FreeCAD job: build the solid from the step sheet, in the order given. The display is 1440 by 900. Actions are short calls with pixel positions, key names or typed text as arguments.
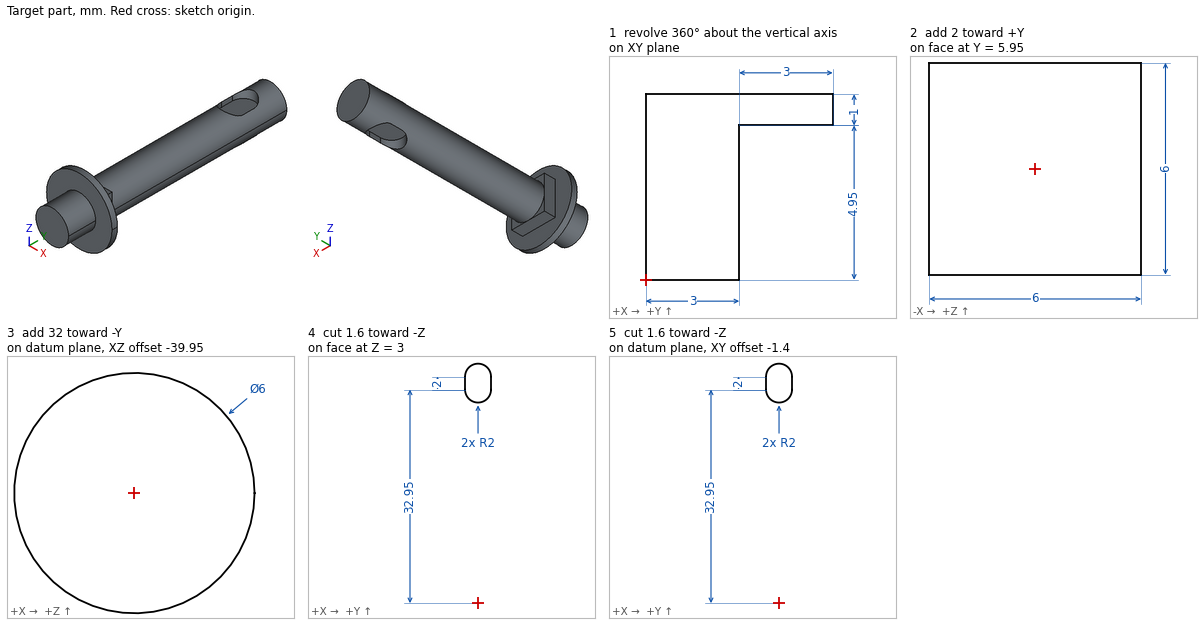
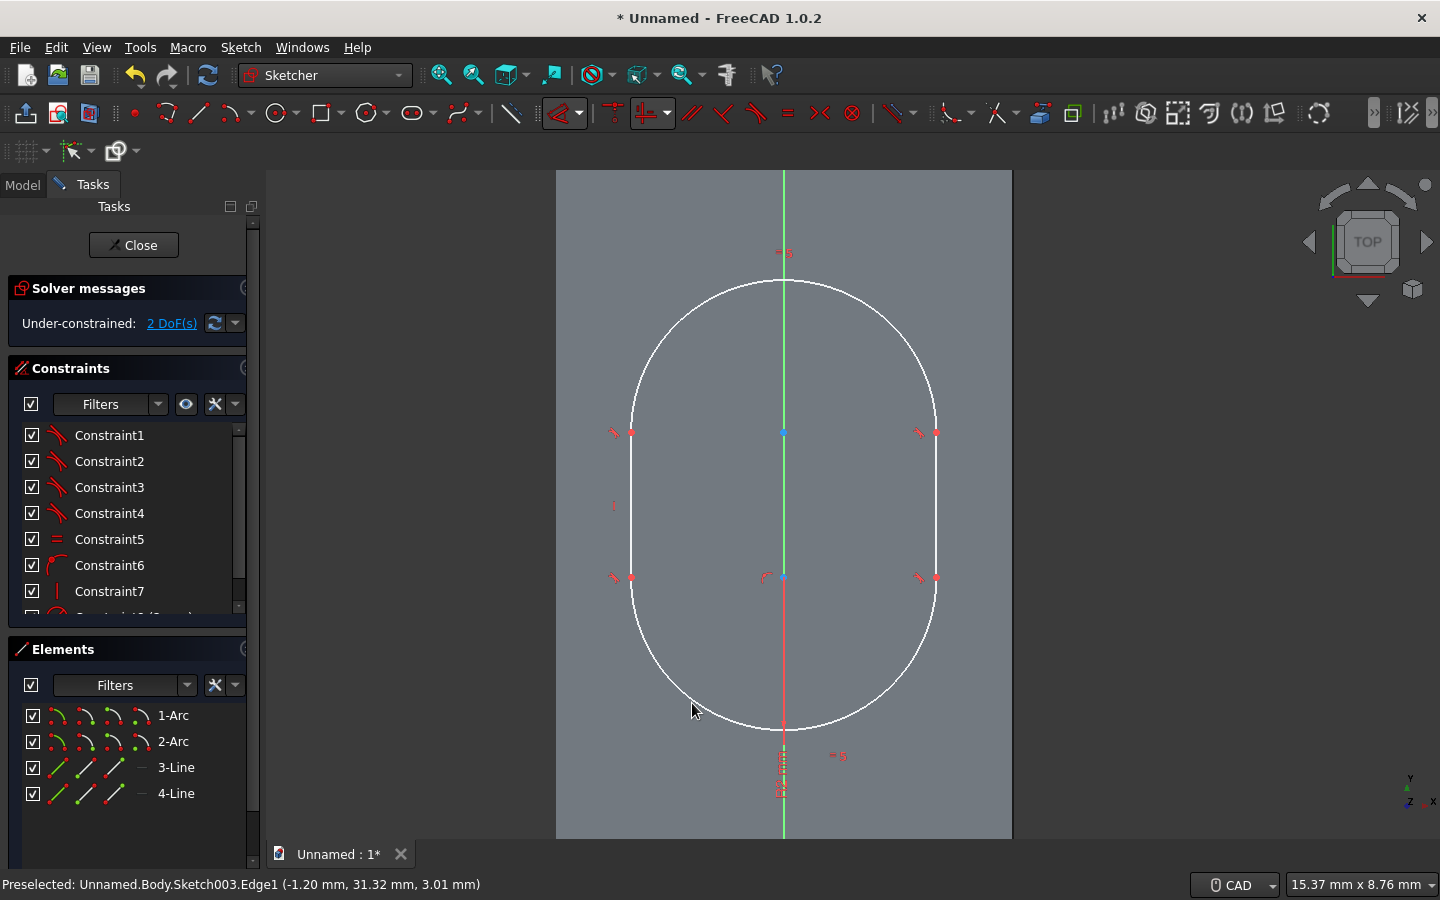
click(631, 534)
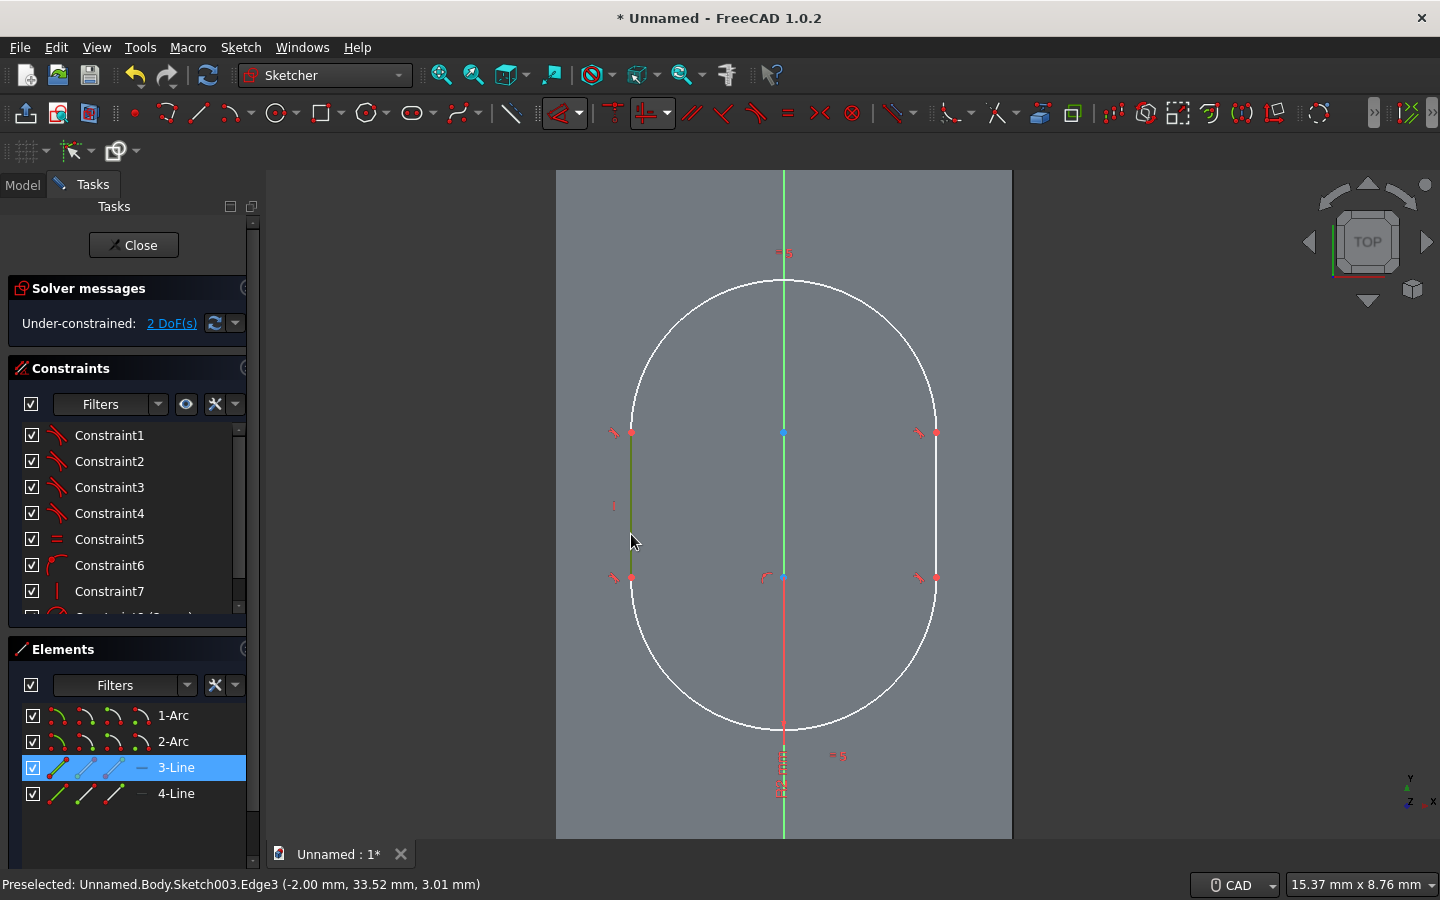
key(i)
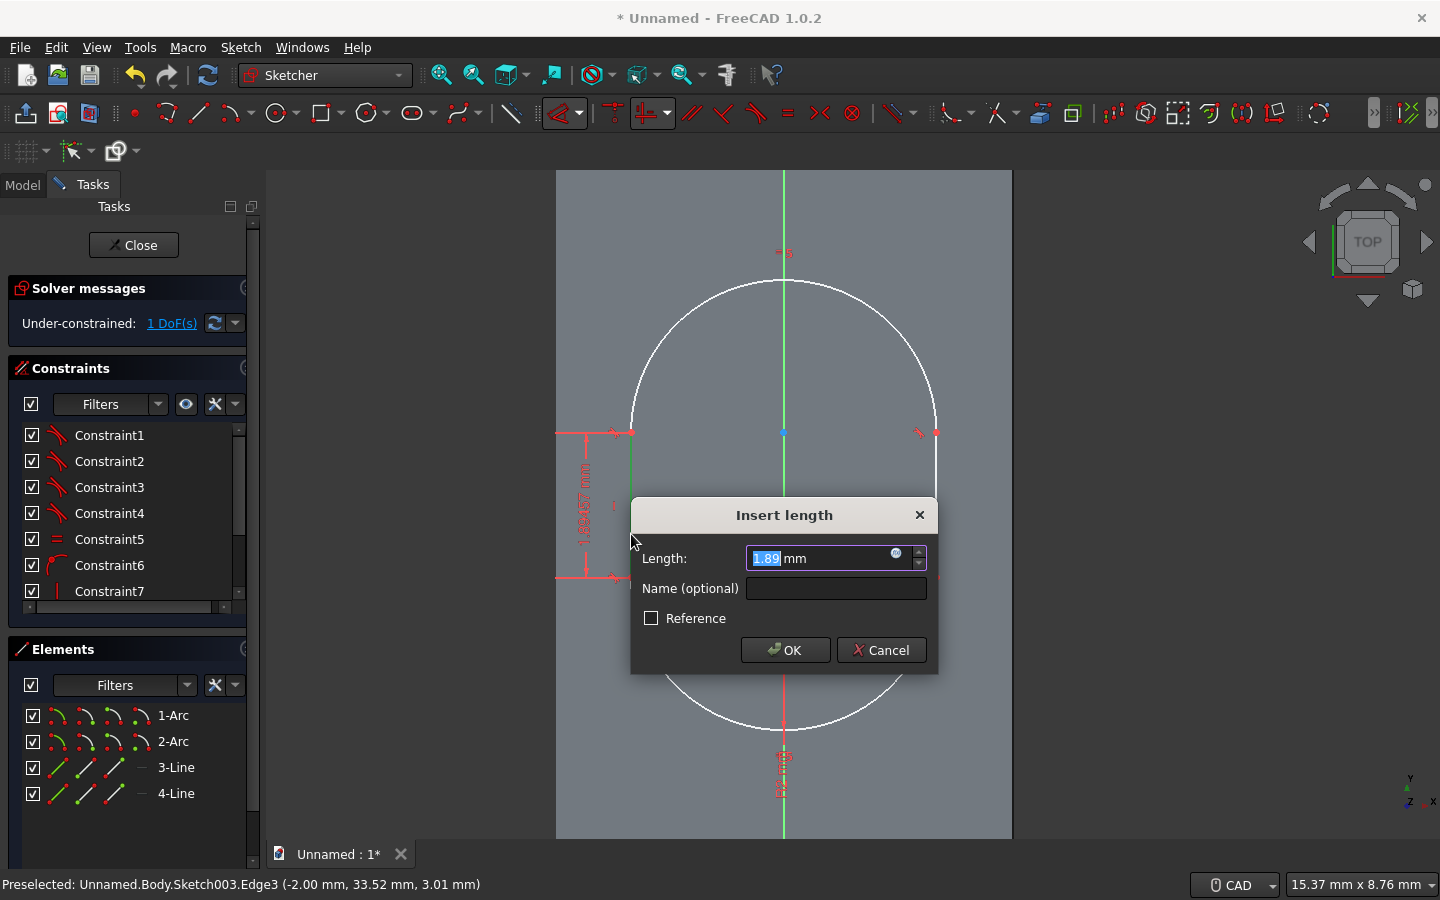
text(2)
key(Return)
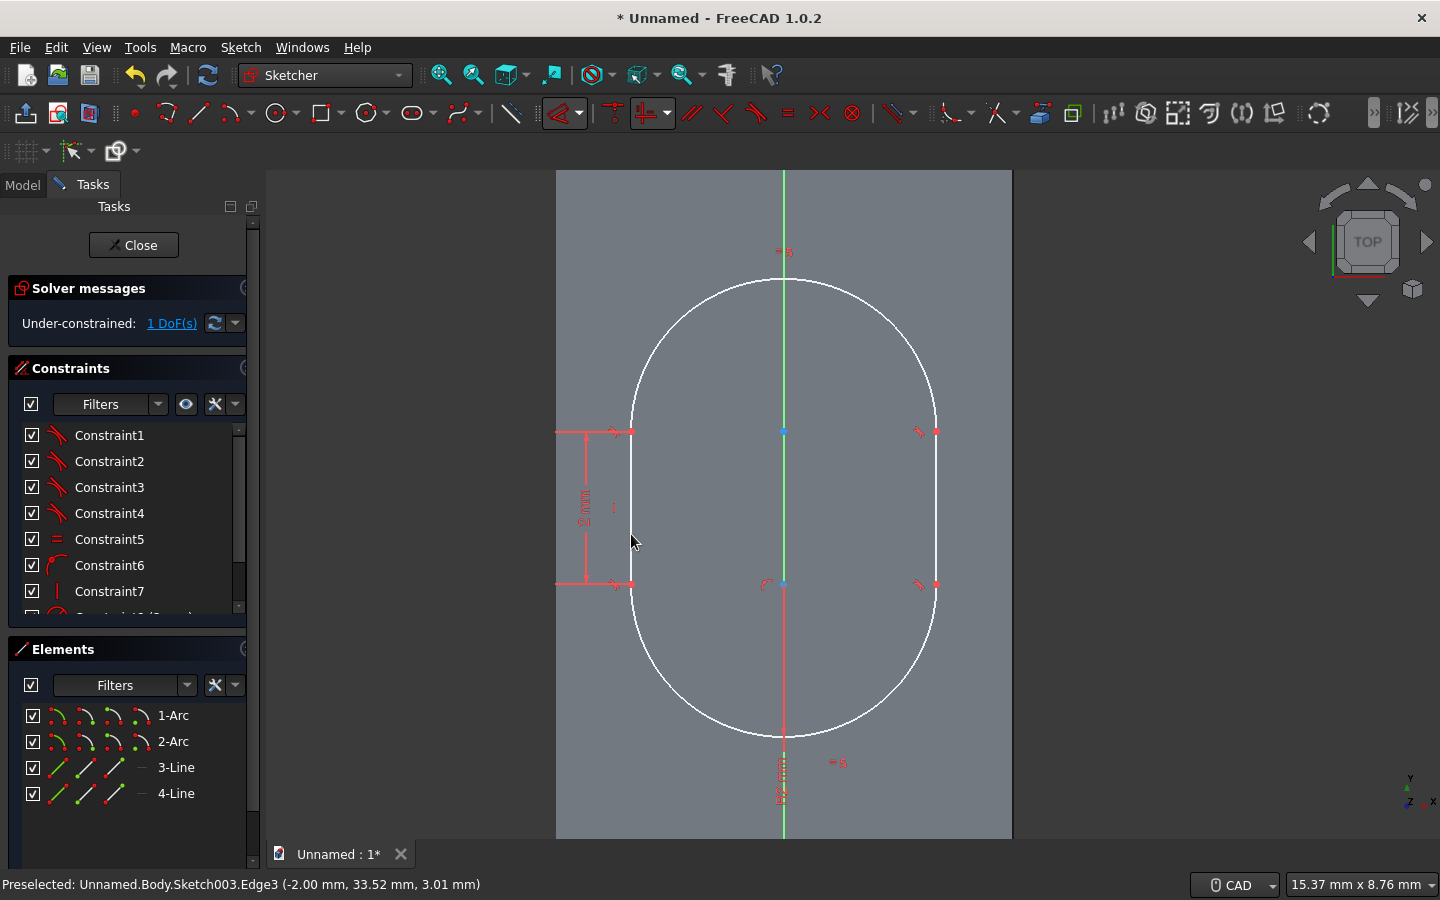
click(631, 584)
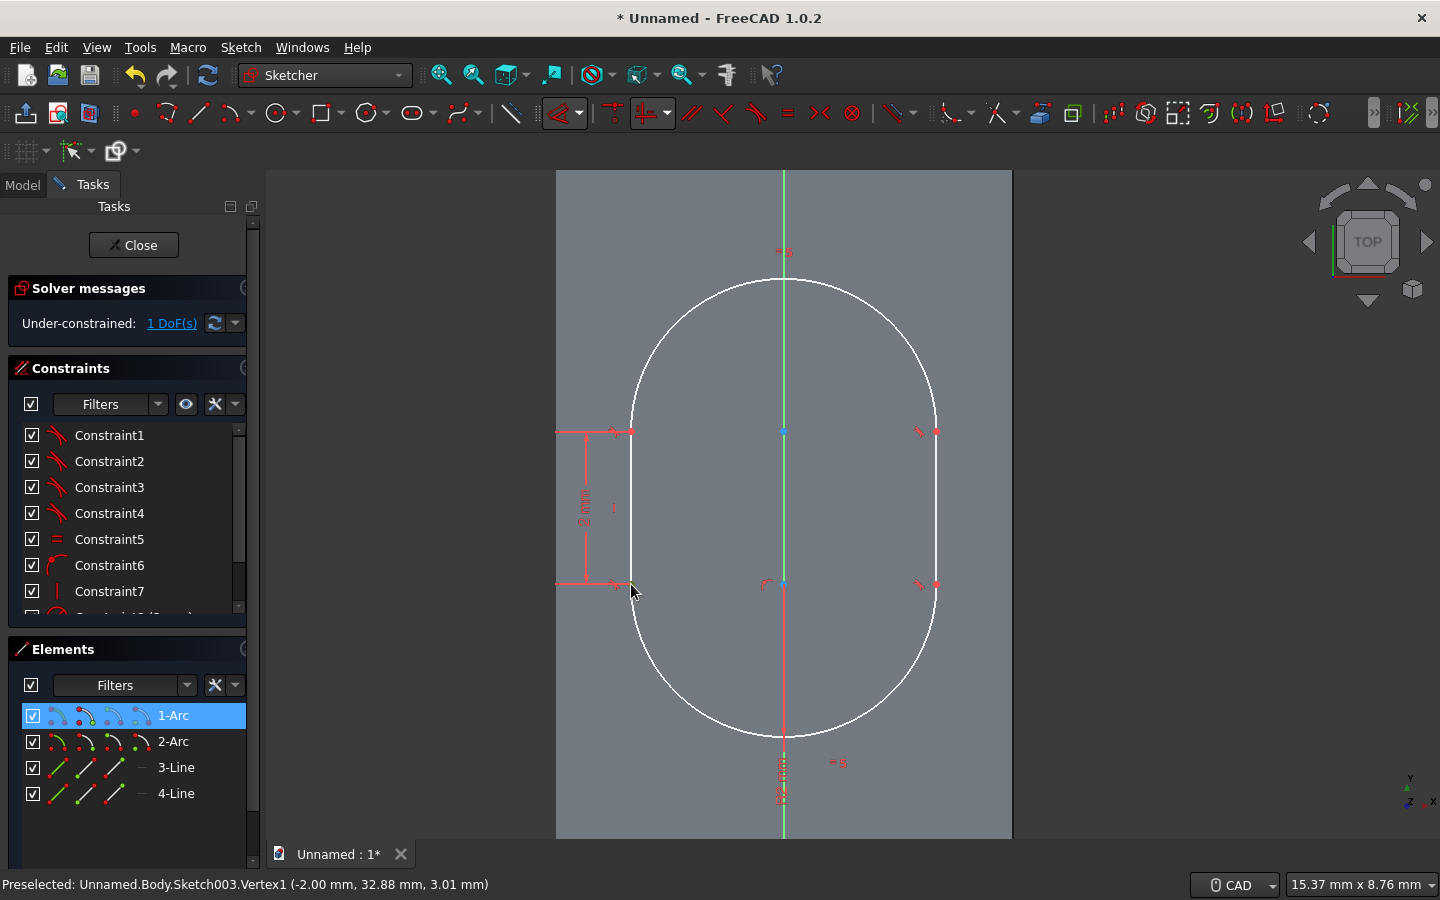
click(582, 114)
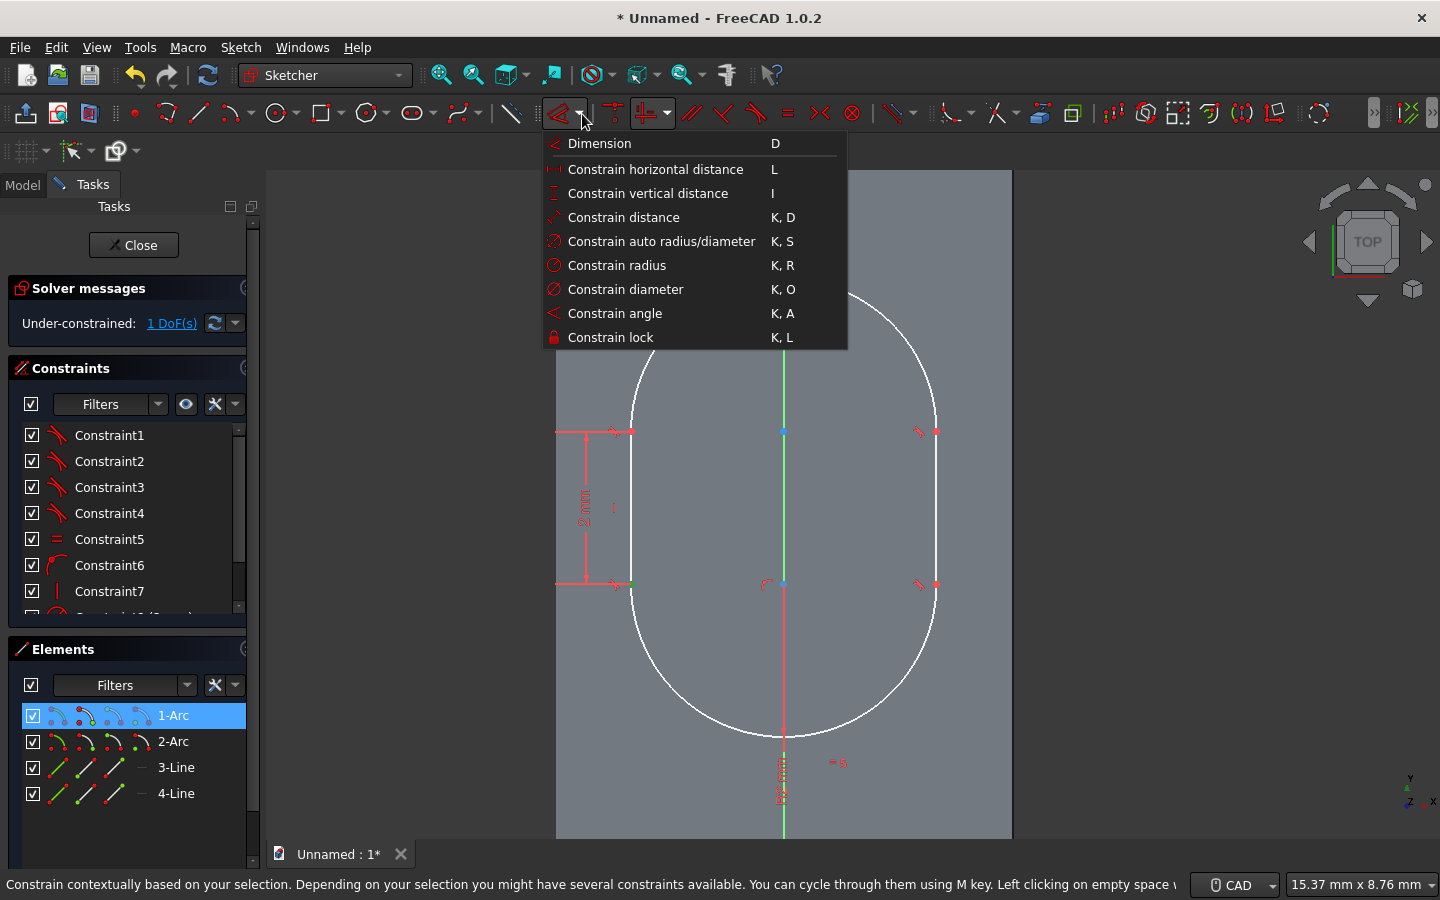
click(695, 193)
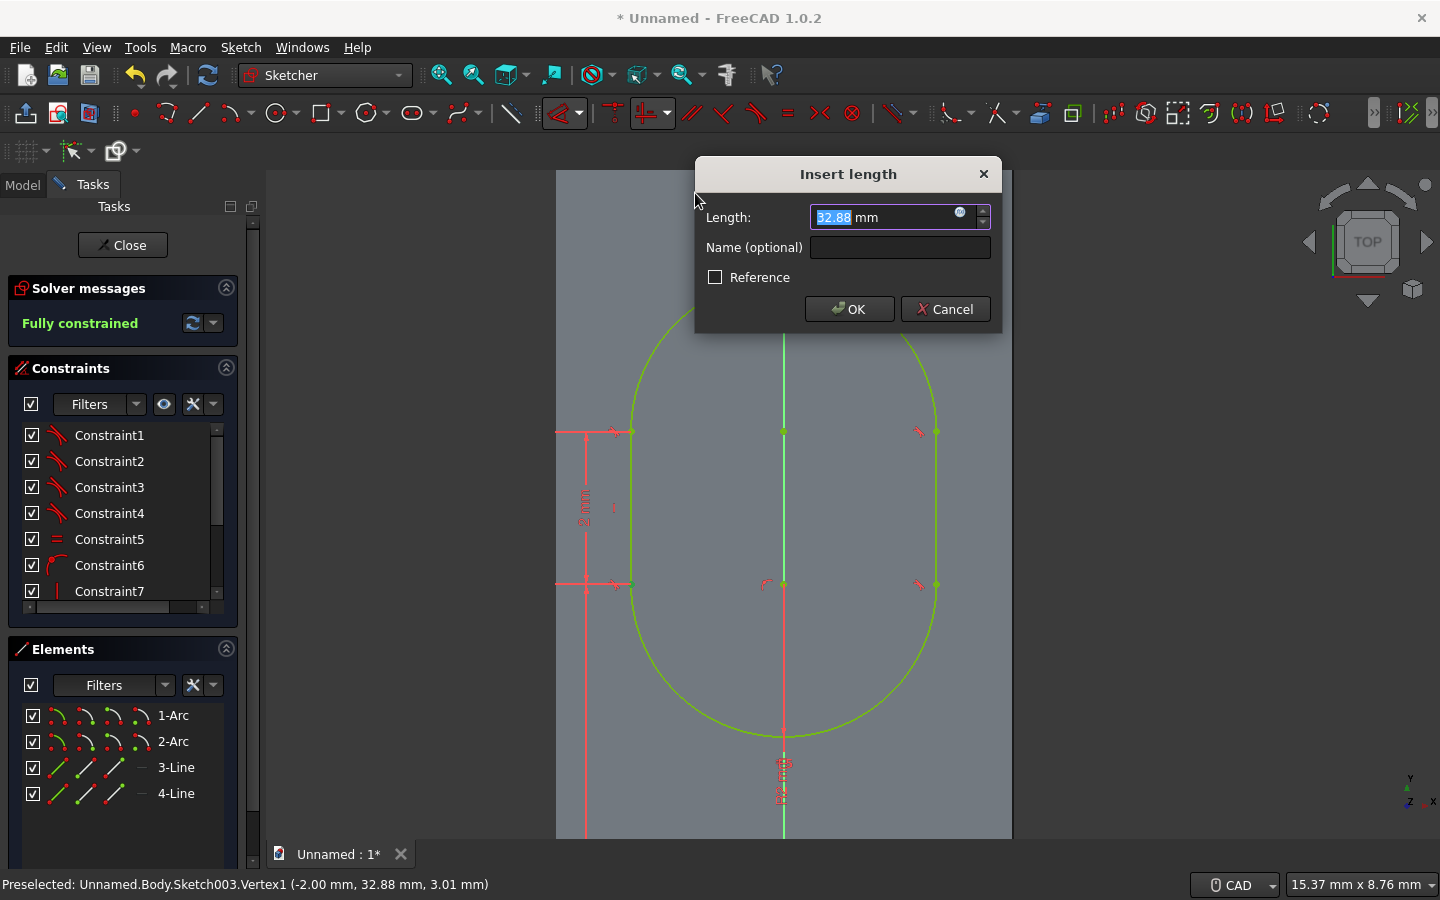
text(32.95)
key(Return)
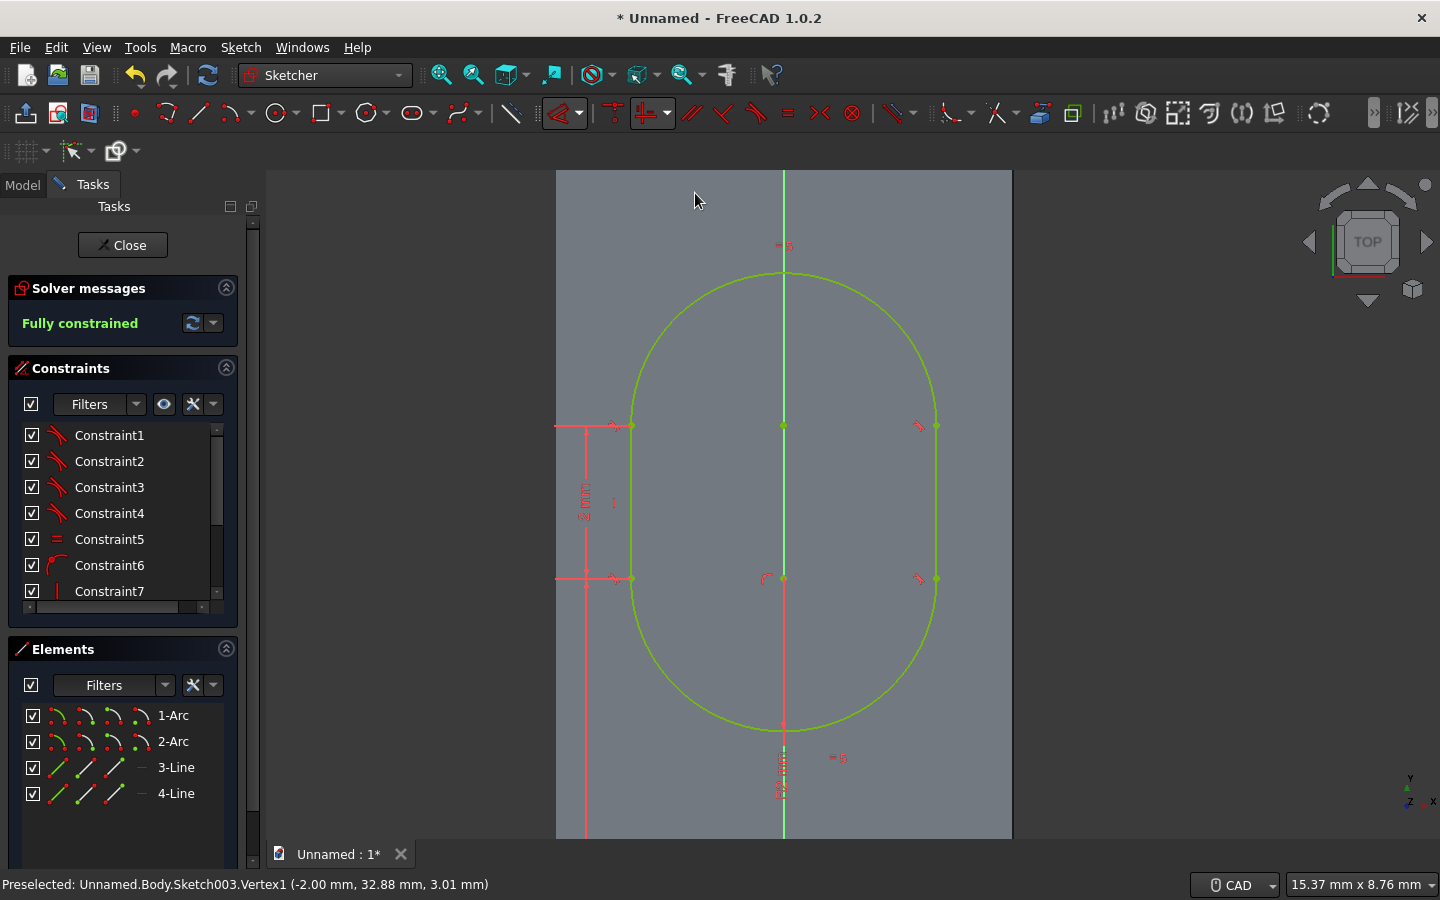
click(123, 245)